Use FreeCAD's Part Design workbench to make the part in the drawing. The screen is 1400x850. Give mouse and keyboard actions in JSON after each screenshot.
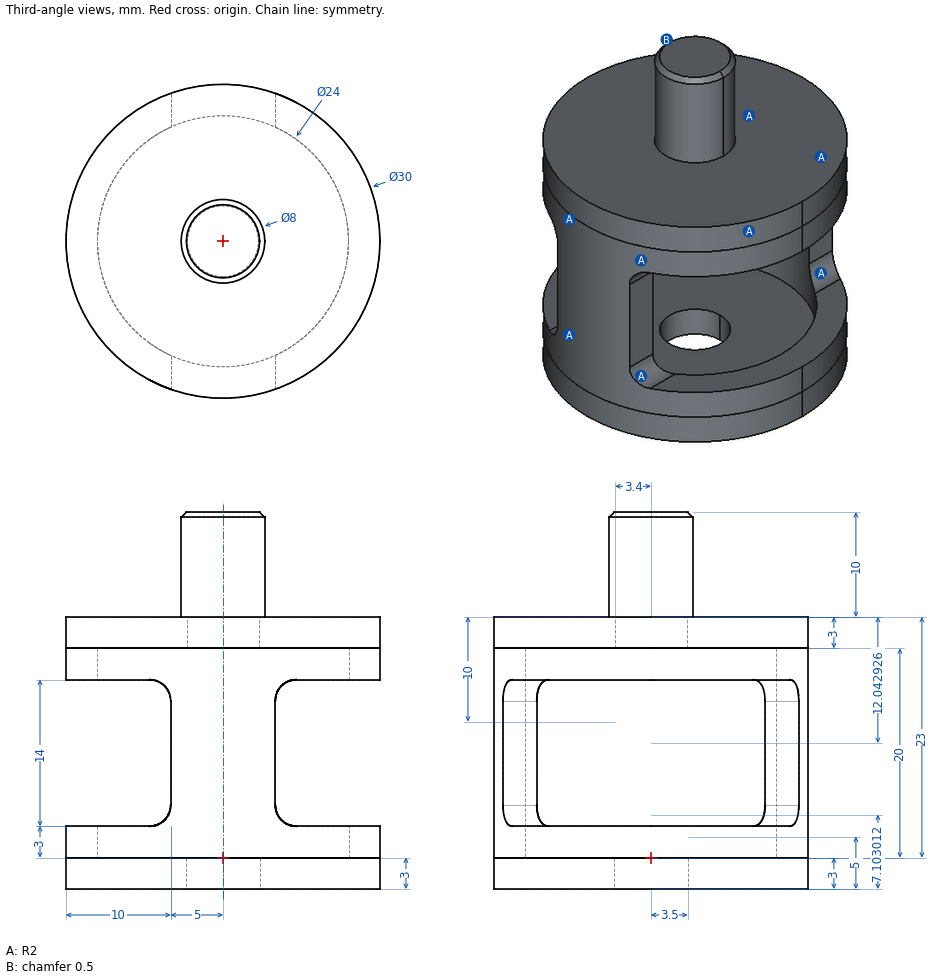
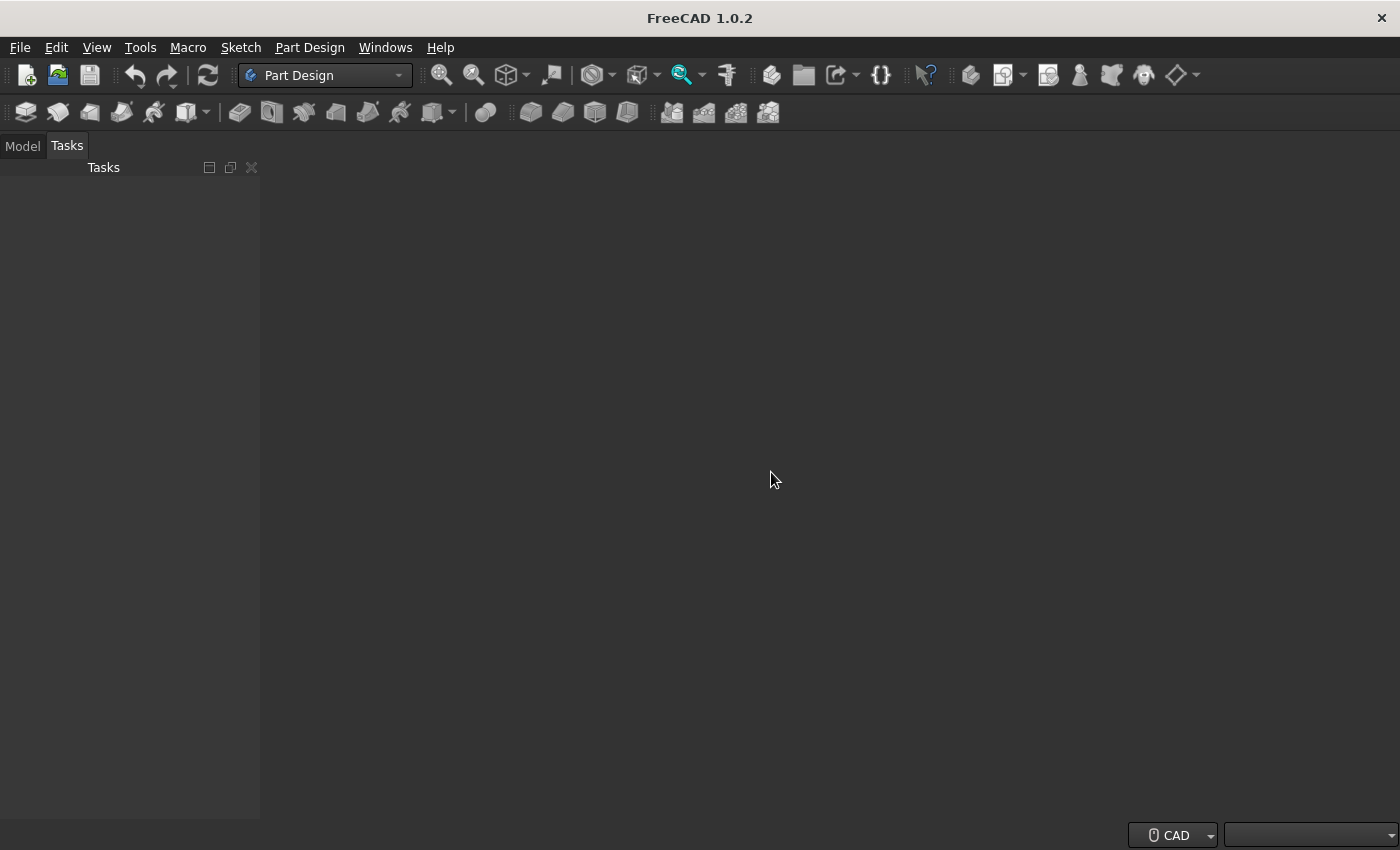
{"action": "left_click", "coordinate": [26, 76]}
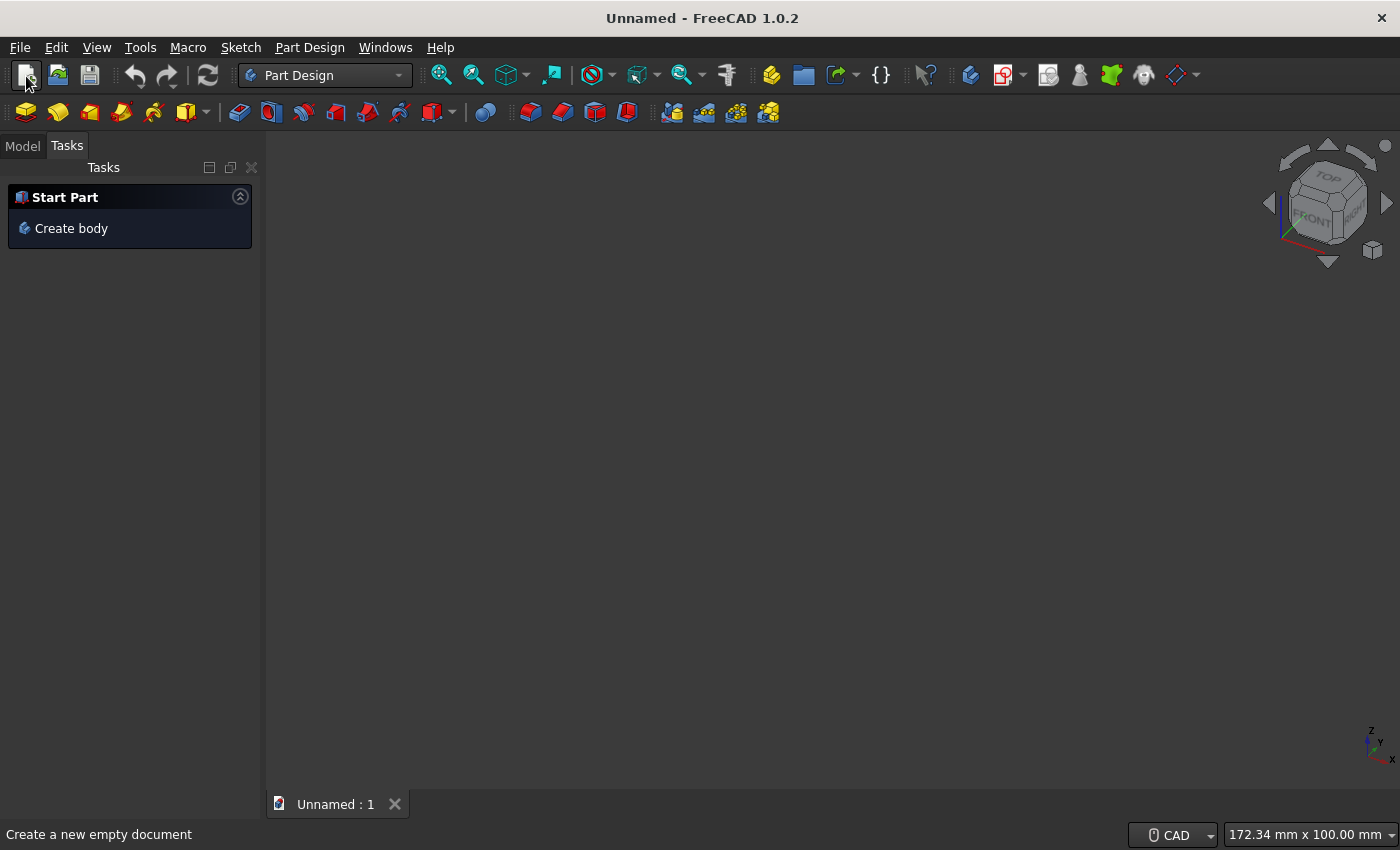
{"action": "left_click", "coordinate": [1004, 76]}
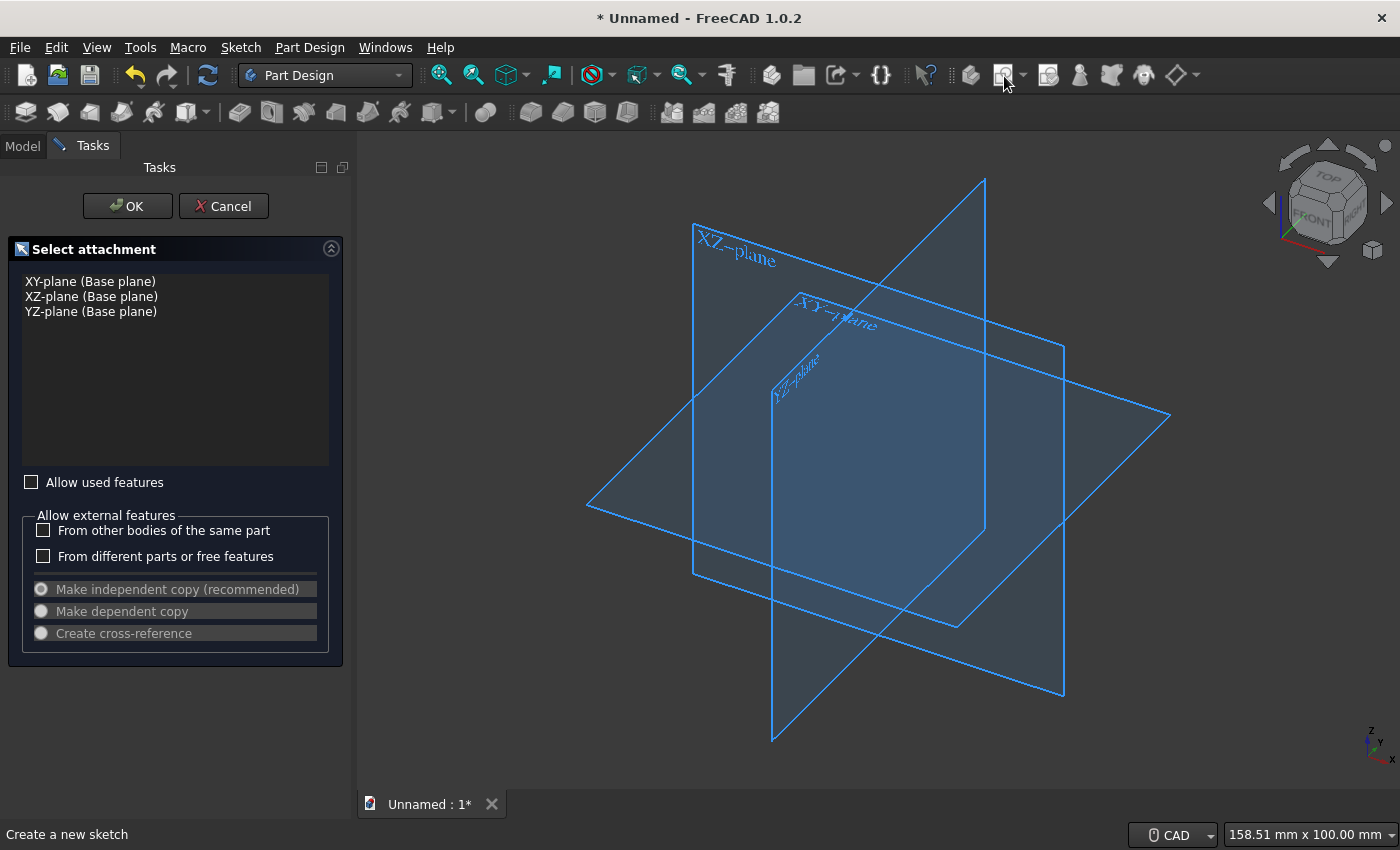
{"action": "left_click", "coordinate": [82, 282]}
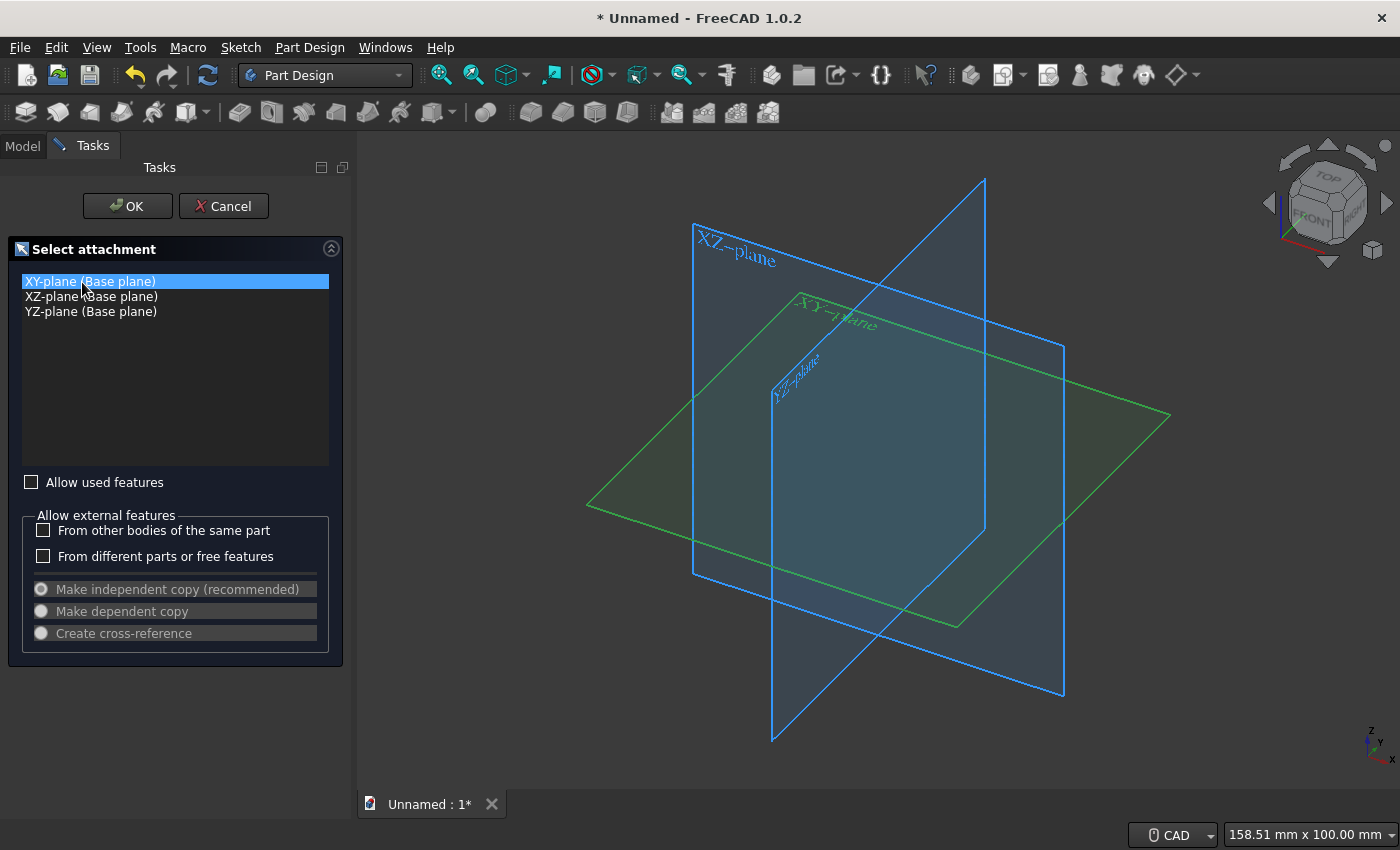
{"action": "left_click", "coordinate": [128, 206]}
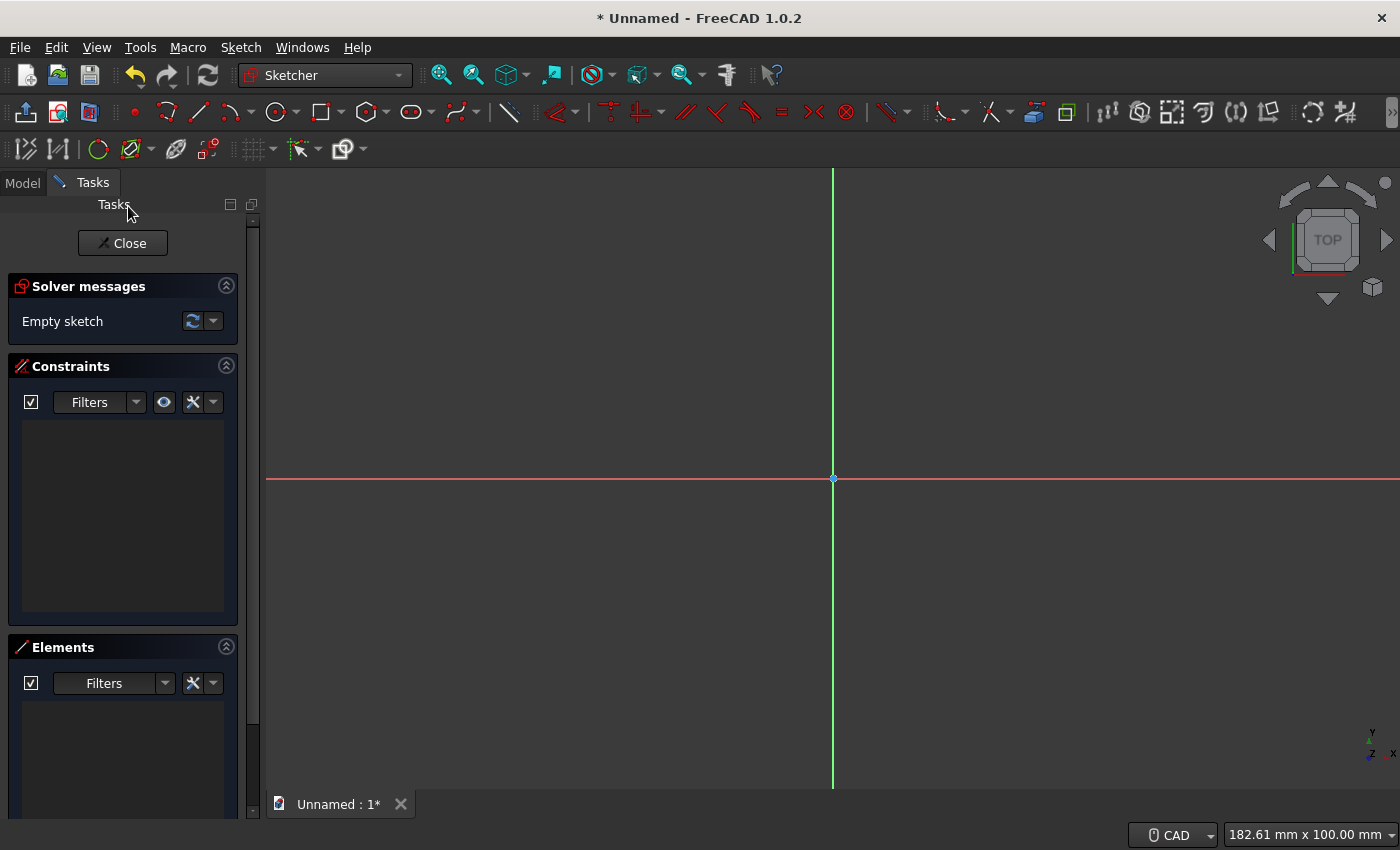
{"action": "scroll", "coordinate": [889, 478], "scroll_direction": "up", "scroll_amount": 4}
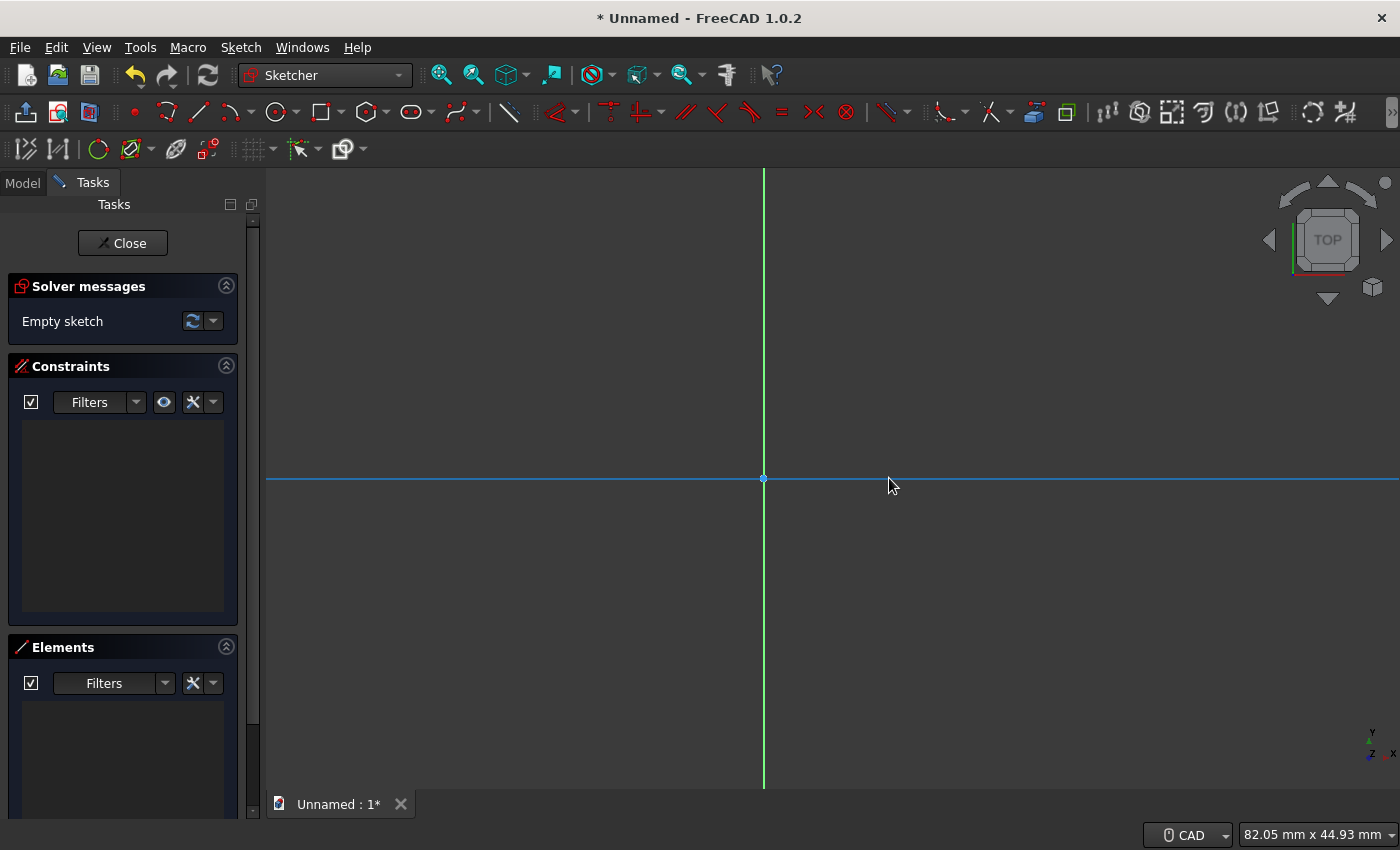
{"action": "key", "text": "g c"}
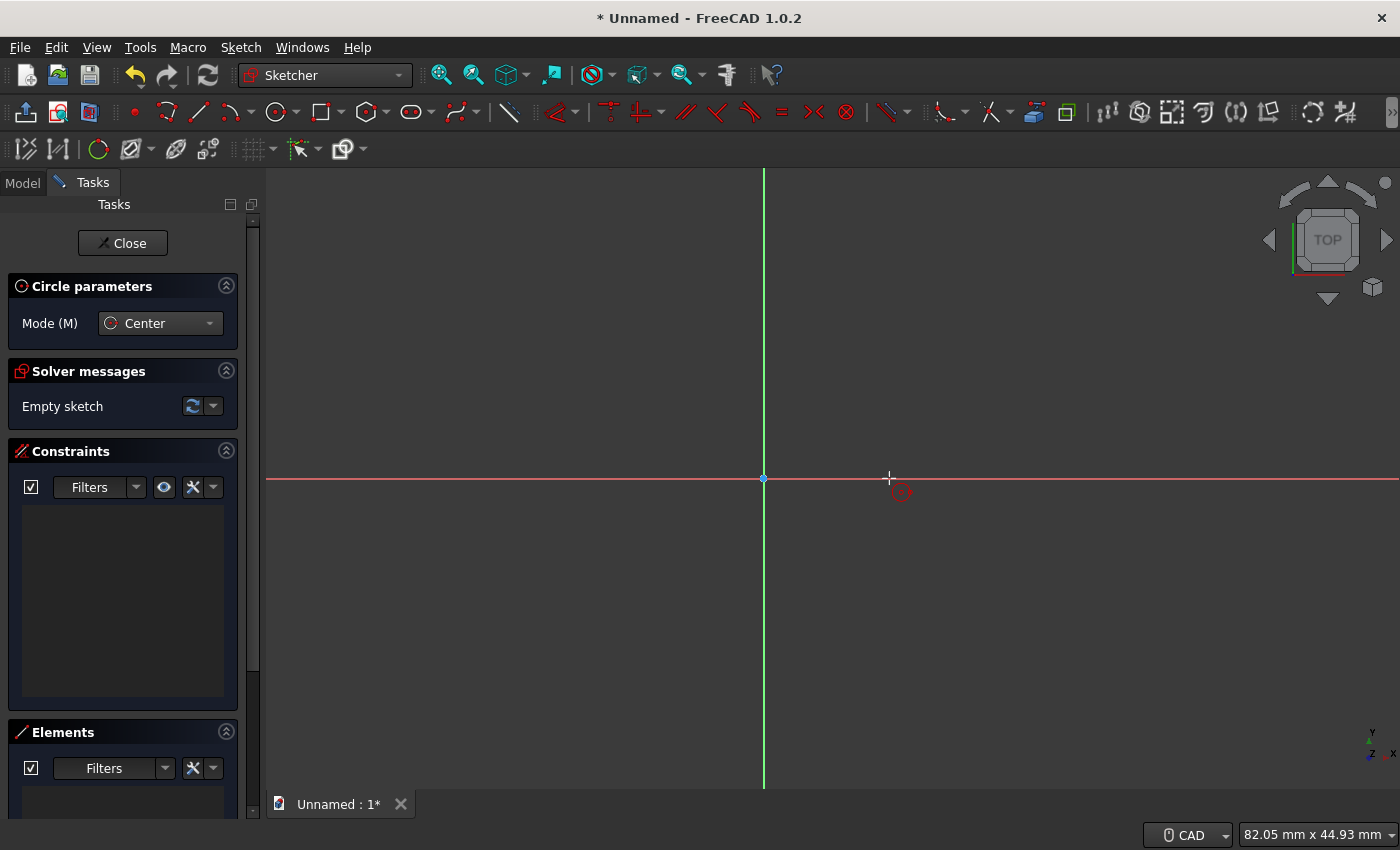
{"action": "left_click", "coordinate": [764, 478]}
{"action": "left_click", "coordinate": [910, 332]}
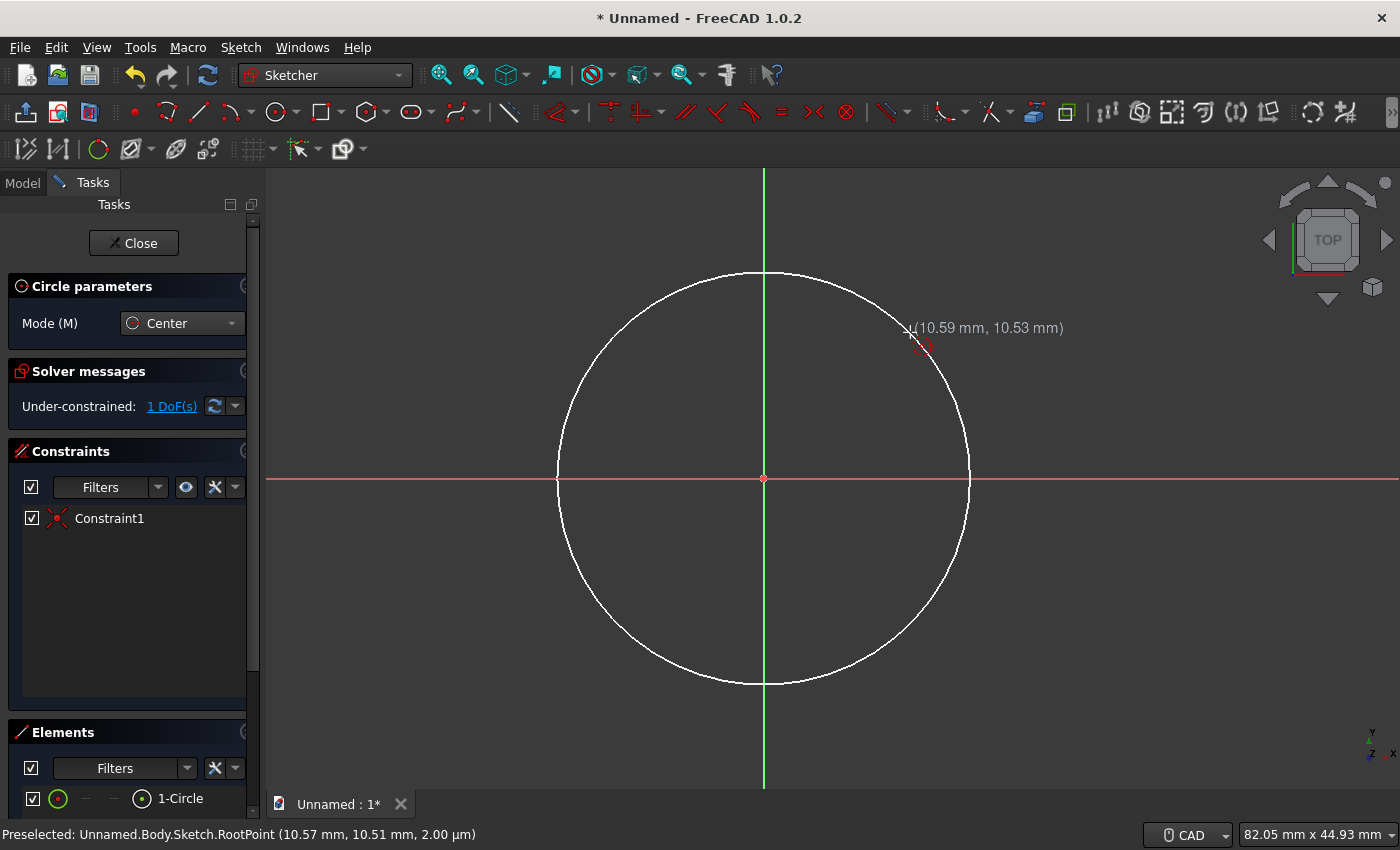
{"action": "left_click", "coordinate": [764, 478]}
{"action": "left_click", "coordinate": [881, 361]}
{"action": "key", "text": "Escape"}